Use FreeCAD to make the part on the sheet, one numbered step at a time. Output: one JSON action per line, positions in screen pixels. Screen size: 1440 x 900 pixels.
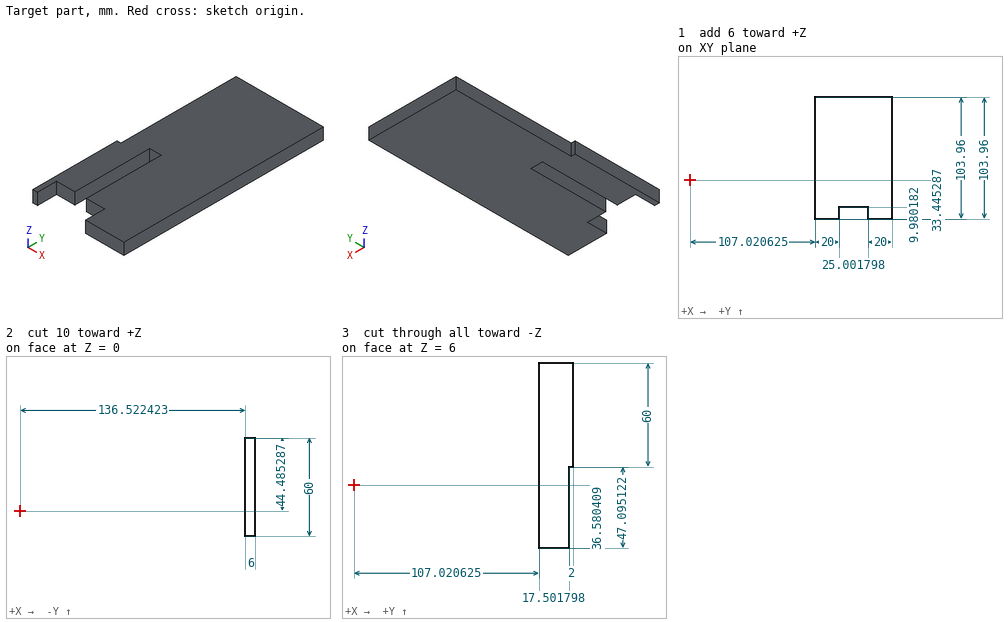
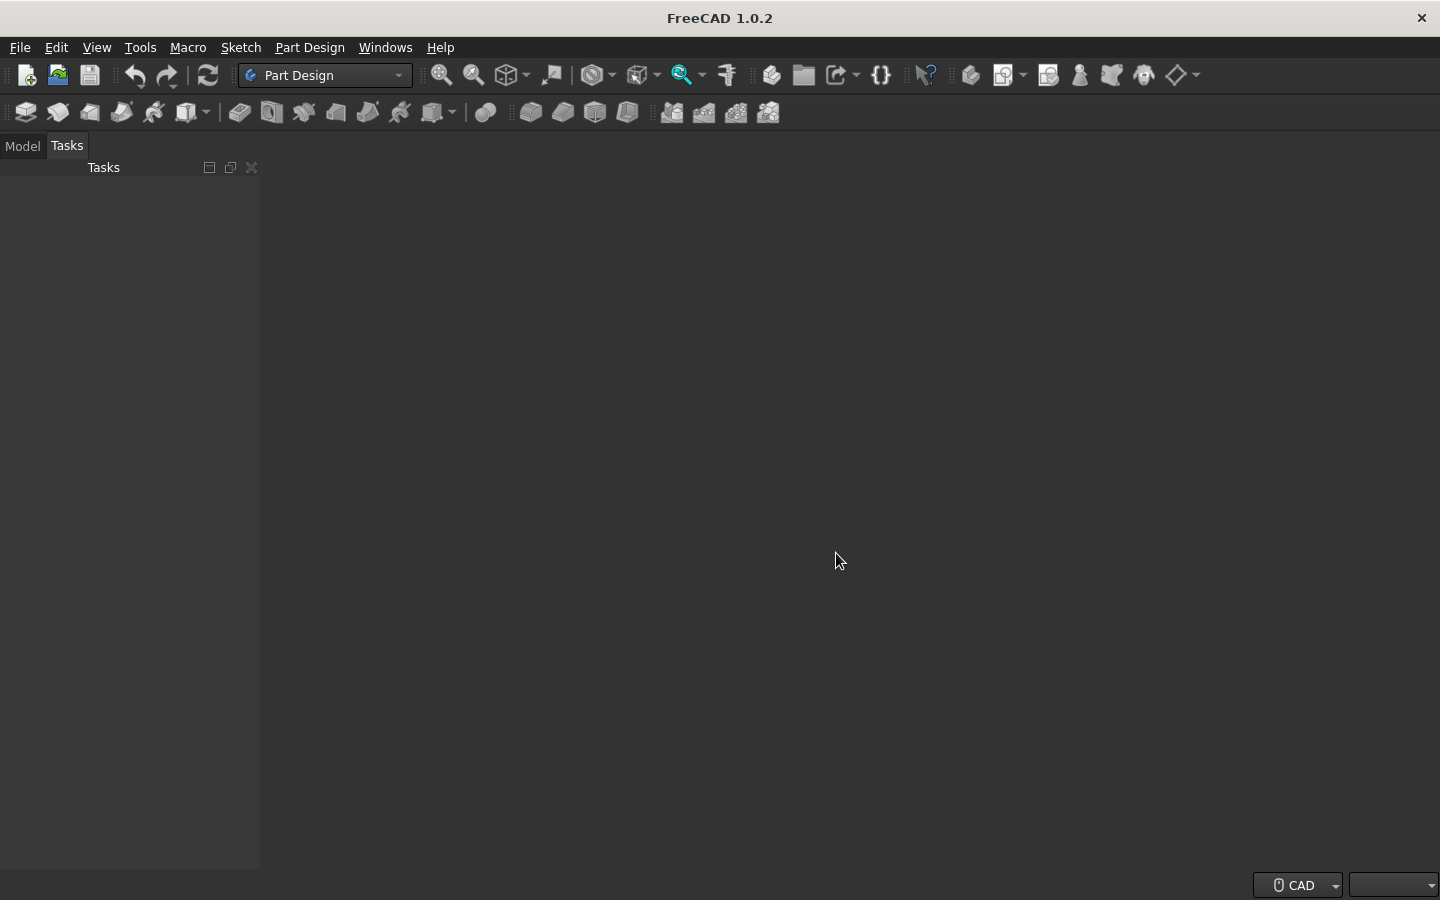
{"action": "left_click", "coordinate": [26, 76]}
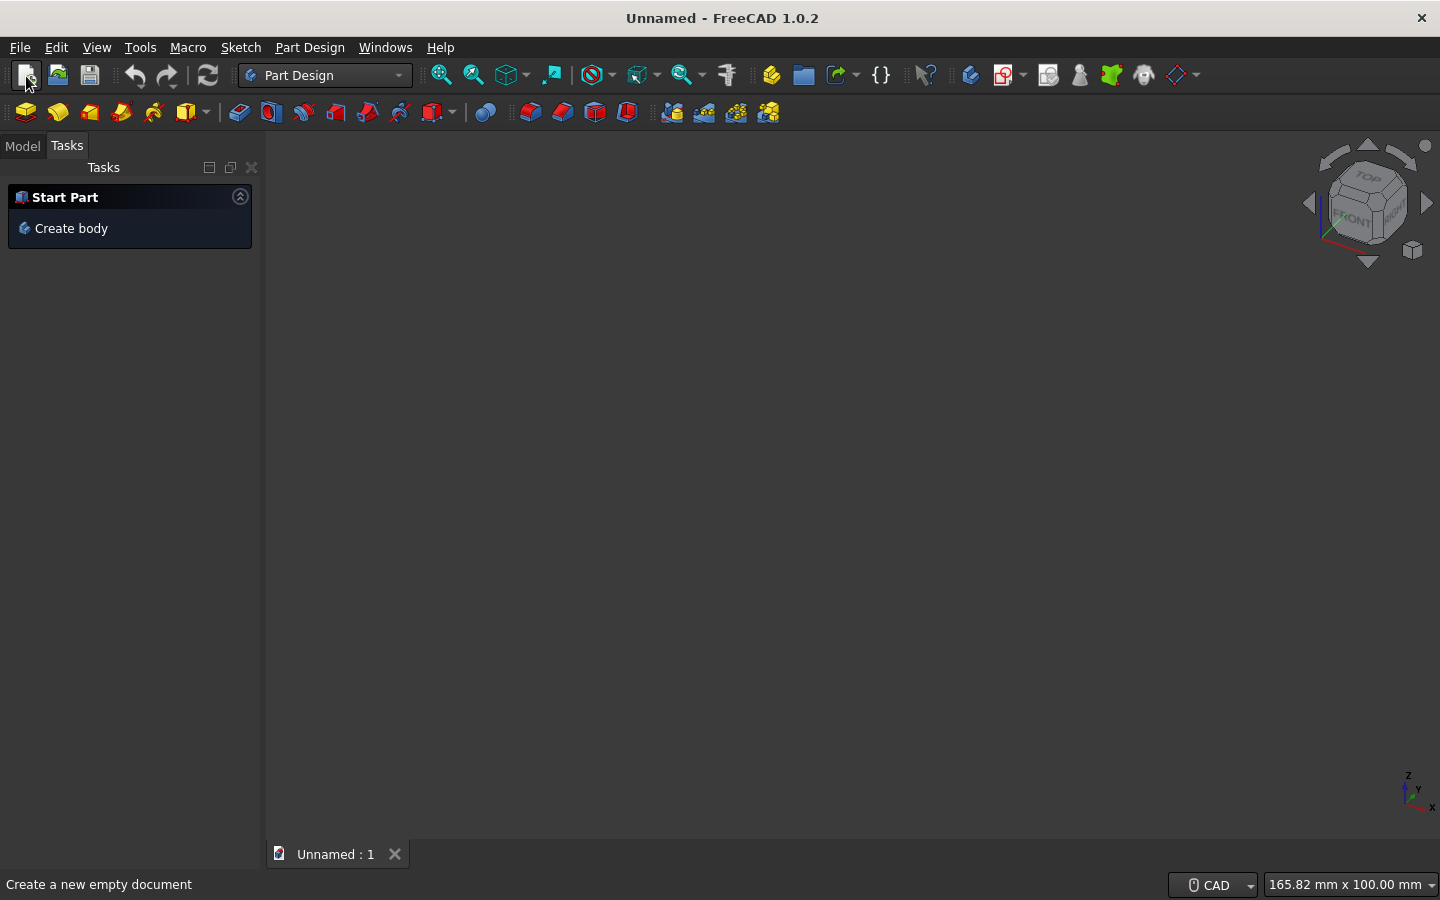
{"action": "left_click", "coordinate": [1004, 76]}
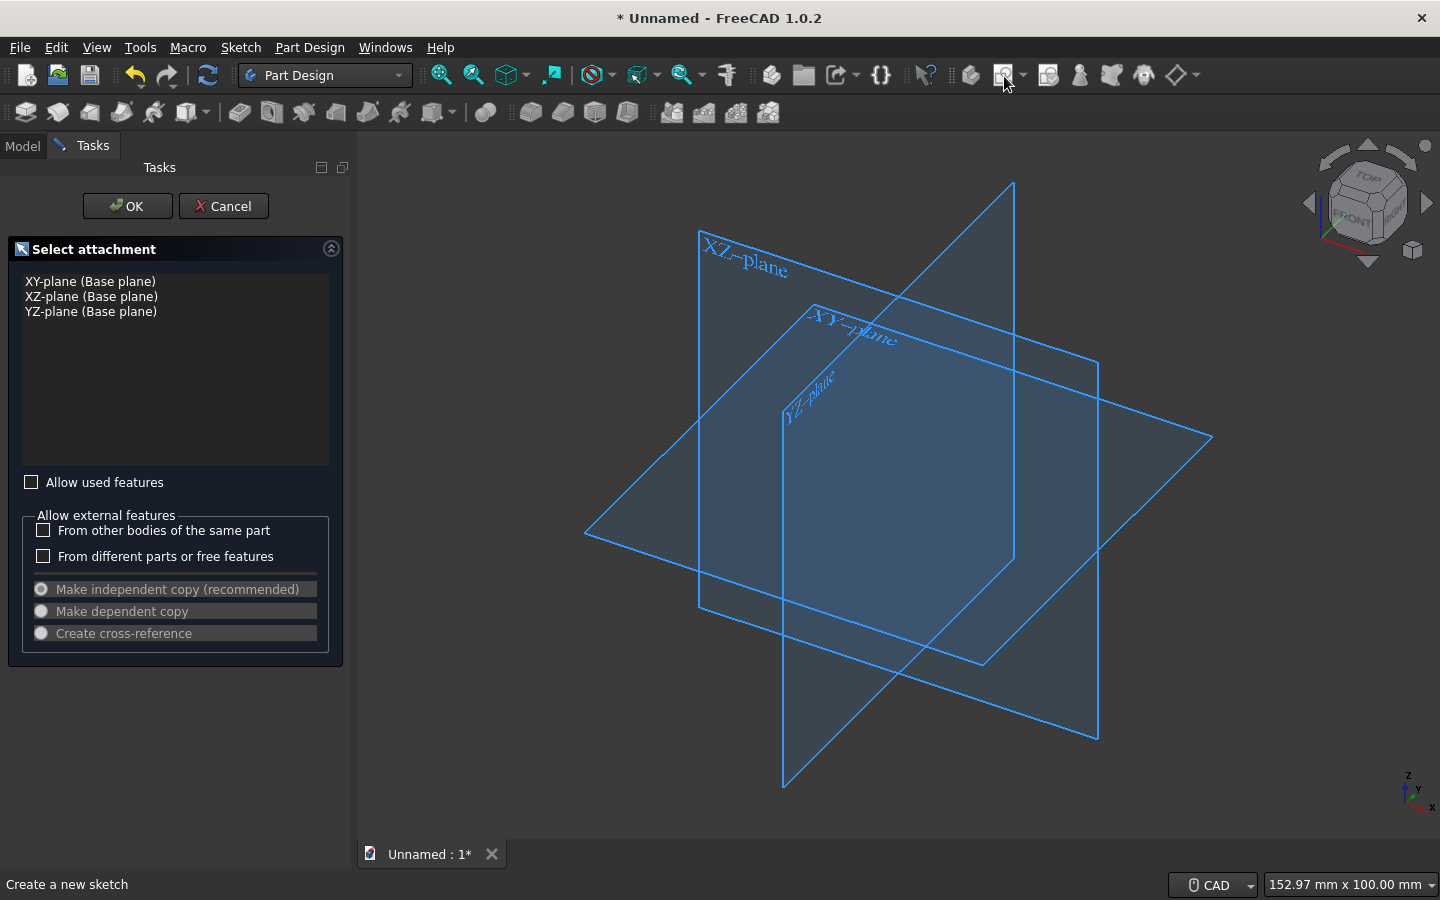
{"action": "left_click", "coordinate": [82, 282]}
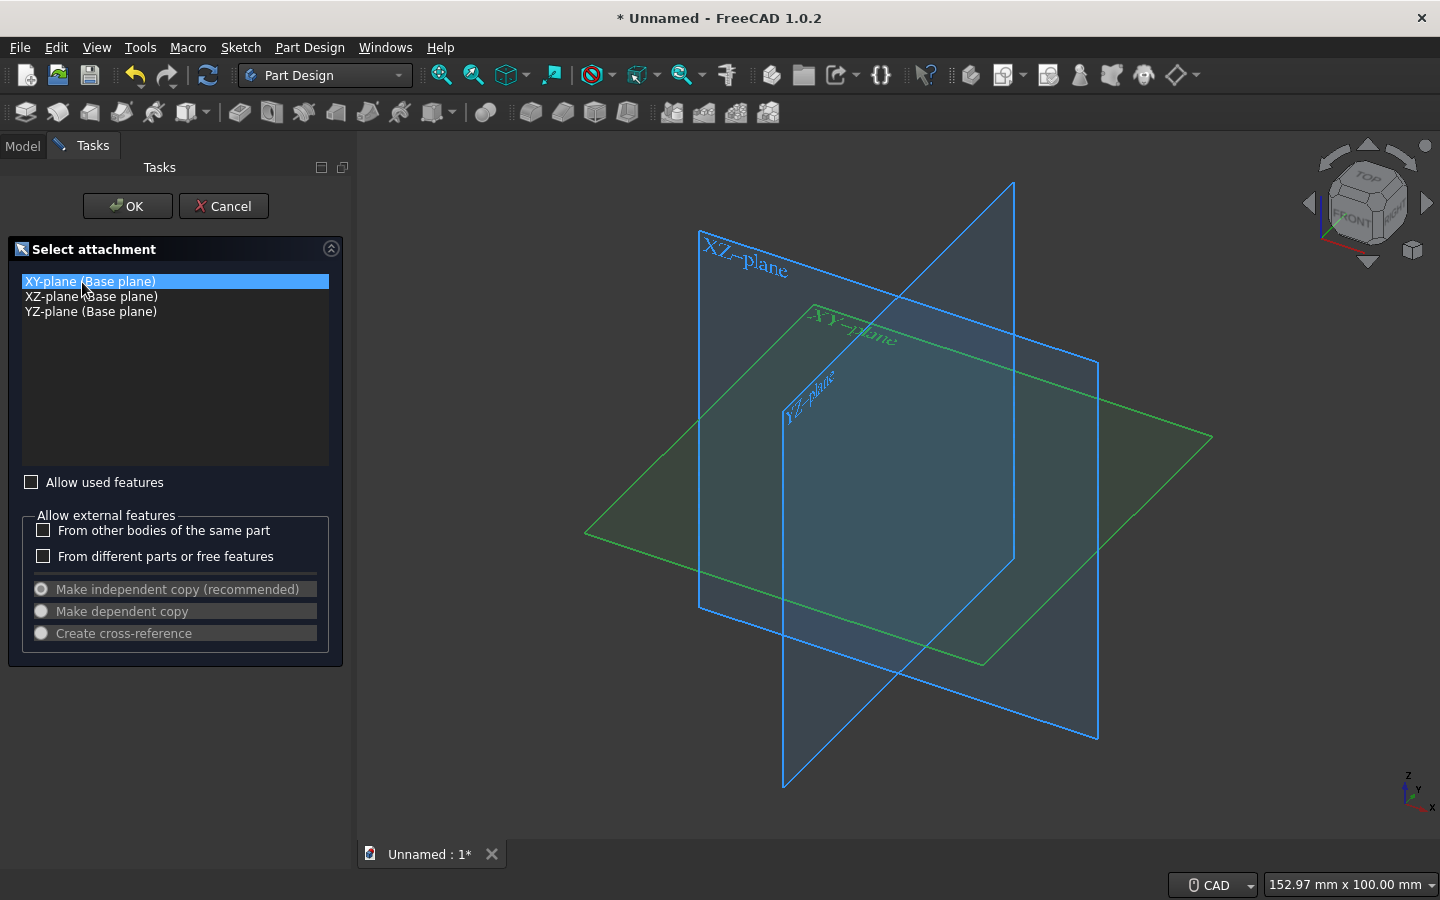
{"action": "left_click", "coordinate": [128, 206]}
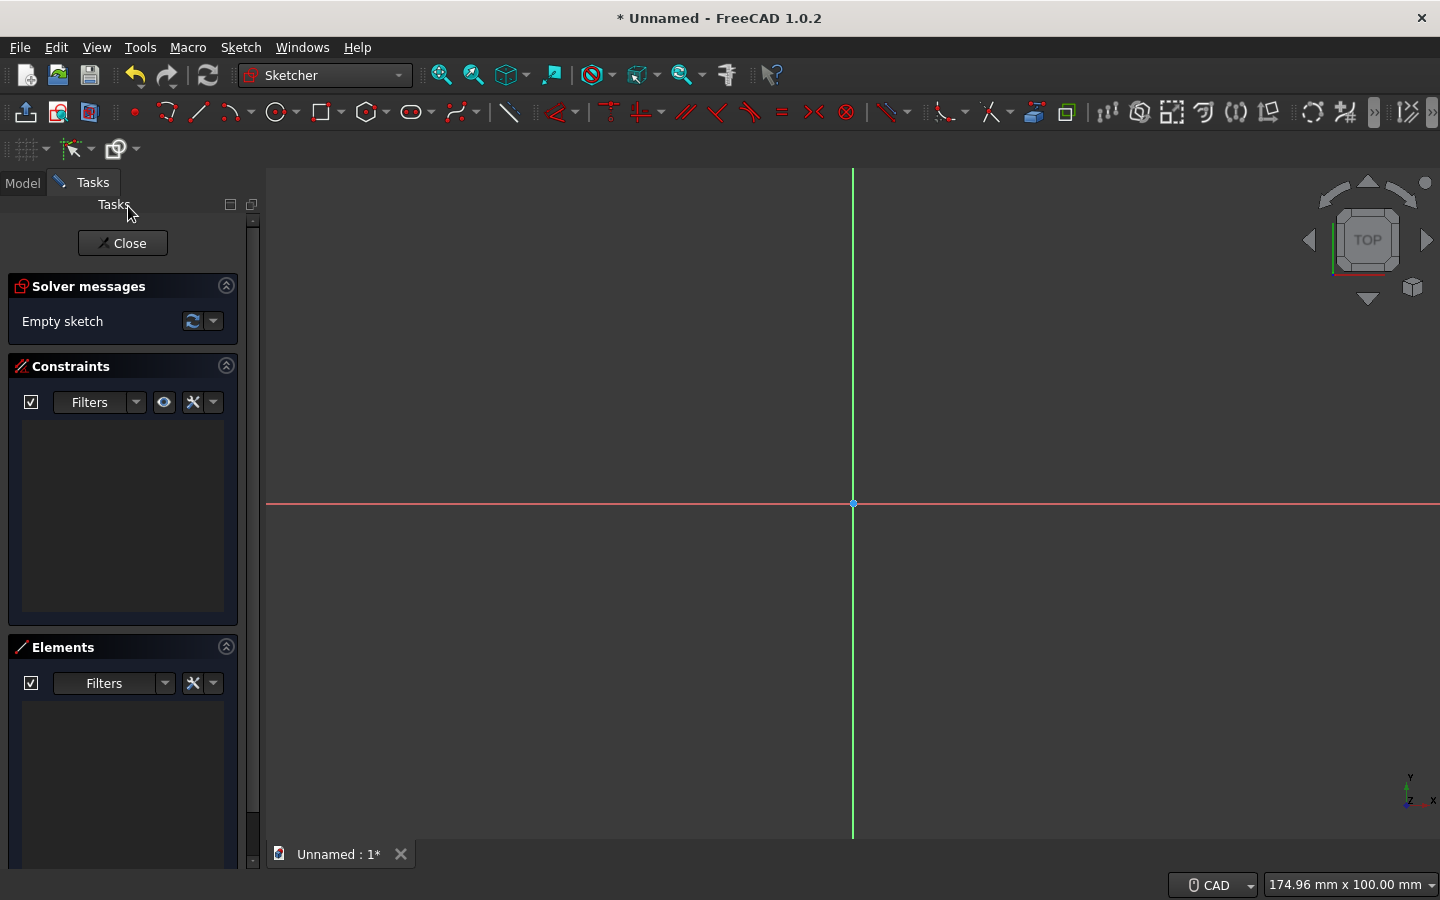
{"action": "scroll", "coordinate": [294, 655], "scroll_direction": "down", "scroll_amount": 3}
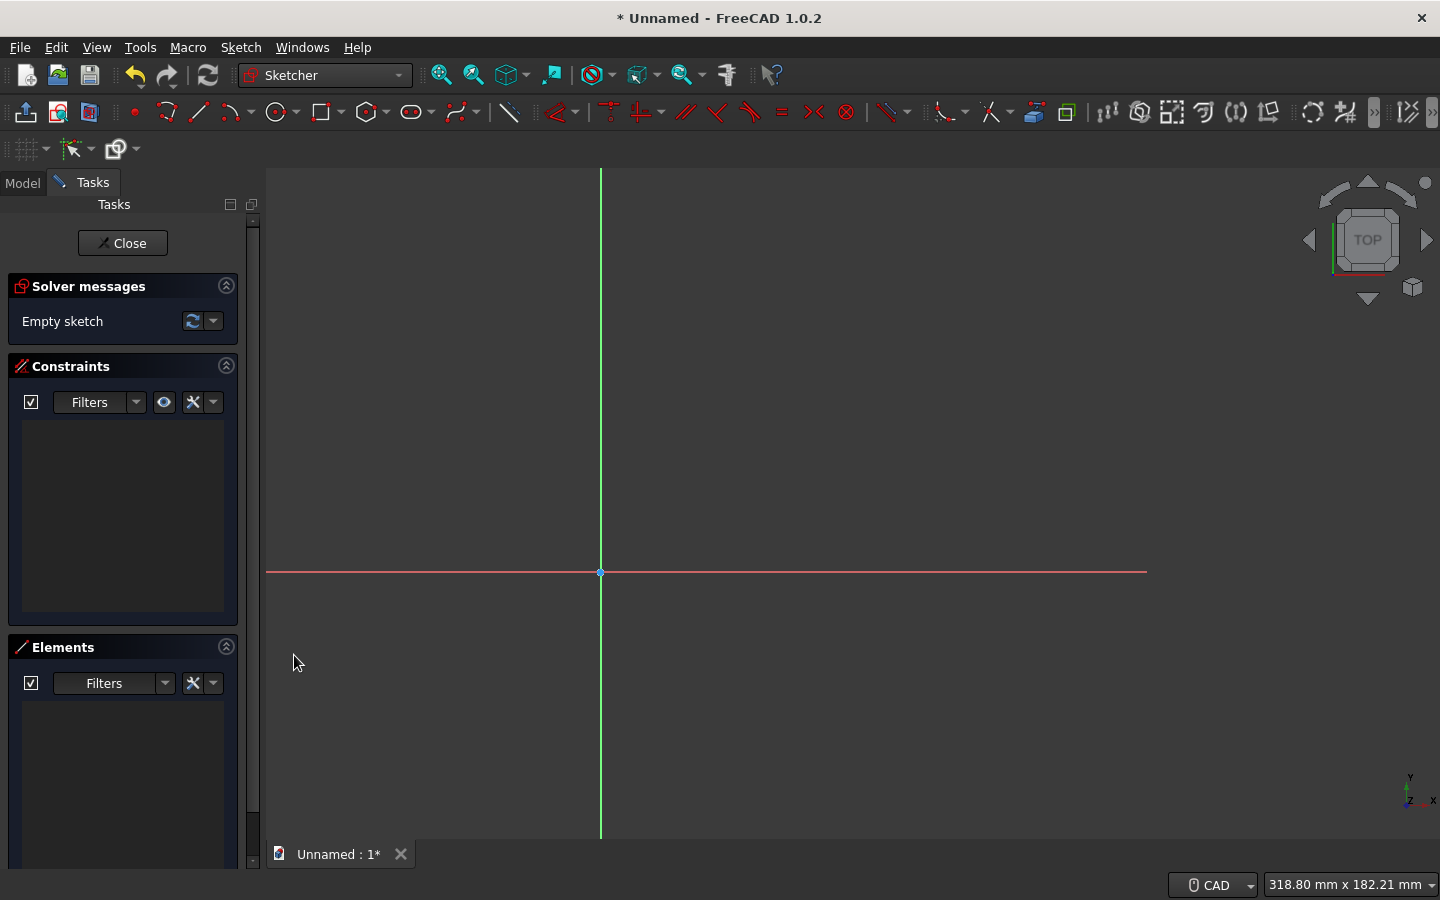
{"action": "left_click", "coordinate": [168, 112]}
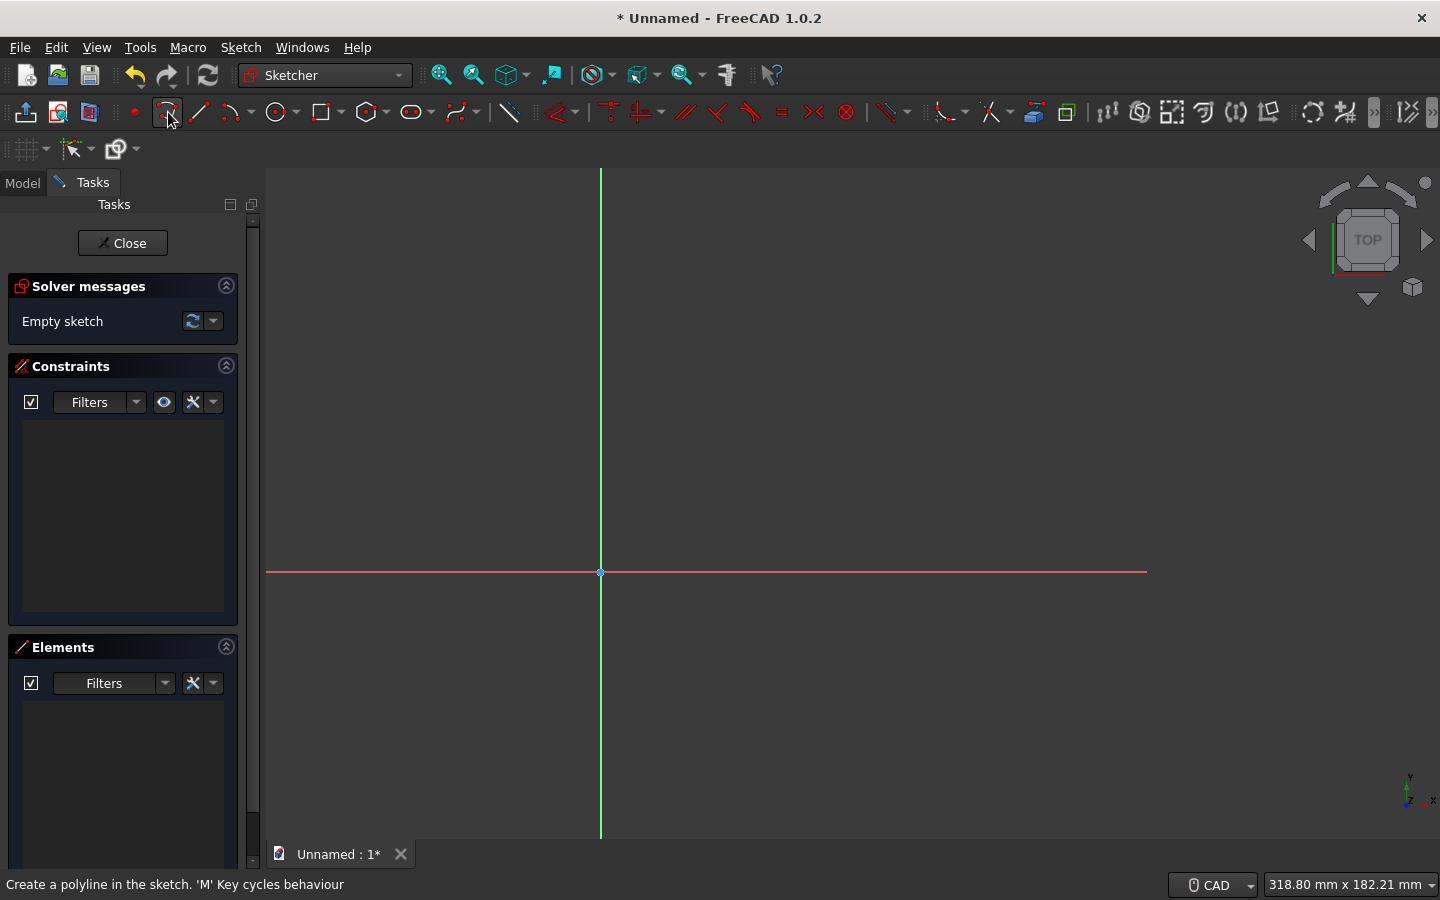
{"action": "left_click", "coordinate": [995, 695]}
{"action": "left_click", "coordinate": [1069, 695]}
{"action": "left_click", "coordinate": [1069, 659]}
{"action": "left_click", "coordinate": [1161, 659]}
{"action": "left_click", "coordinate": [1161, 695]}
{"action": "left_click", "coordinate": [1234, 695]}
{"action": "left_click", "coordinate": [1234, 313]}
{"action": "left_click", "coordinate": [995, 313]}
{"action": "left_click", "coordinate": [995, 696]}
{"action": "key", "text": "Escape"}
{"action": "key", "text": "Escape"}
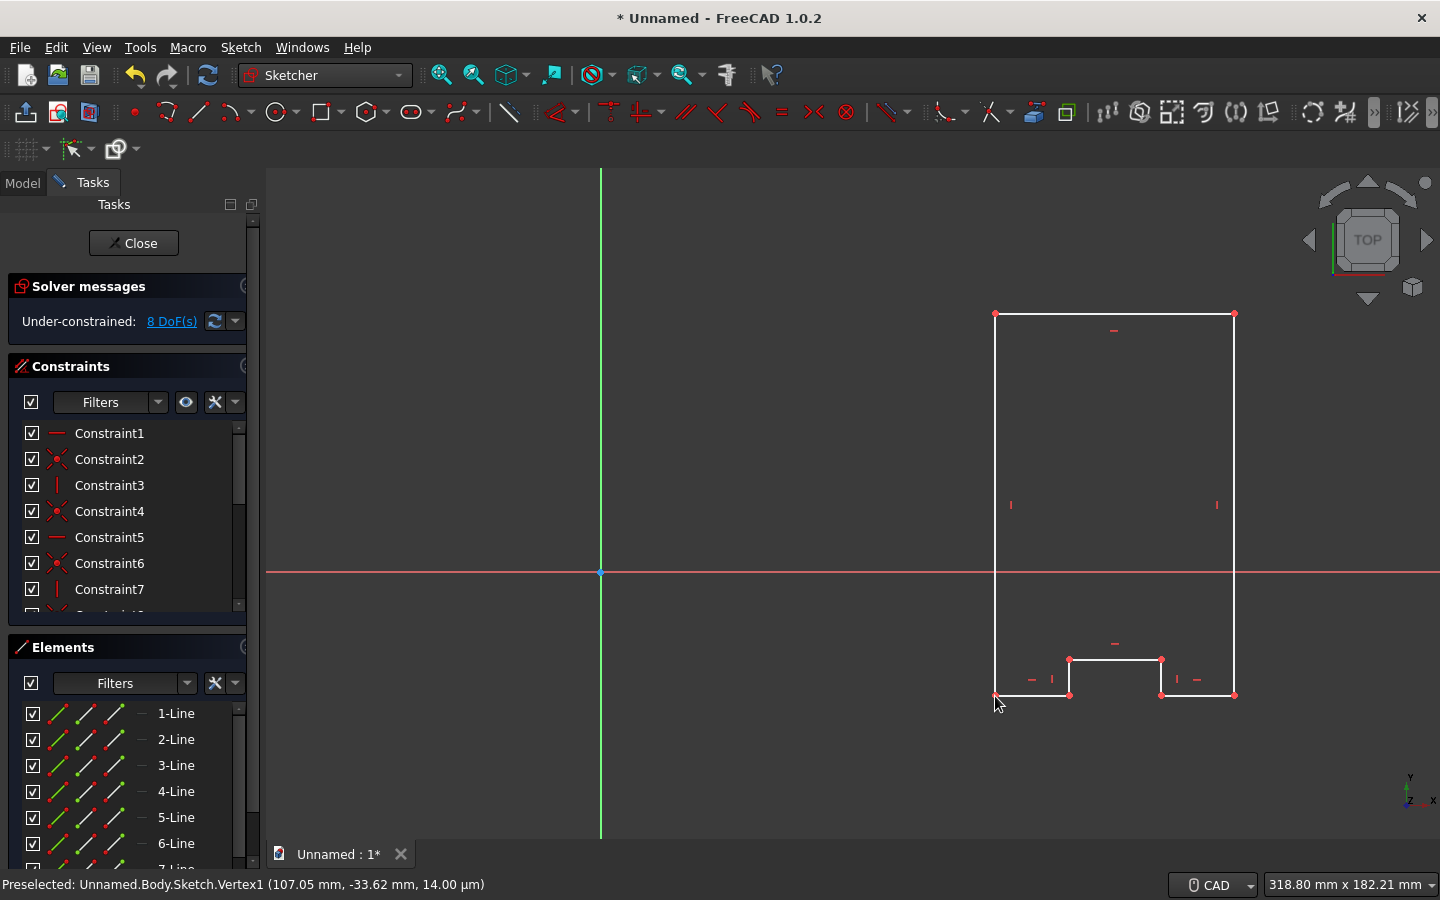
{"action": "left_click", "coordinate": [556, 112]}